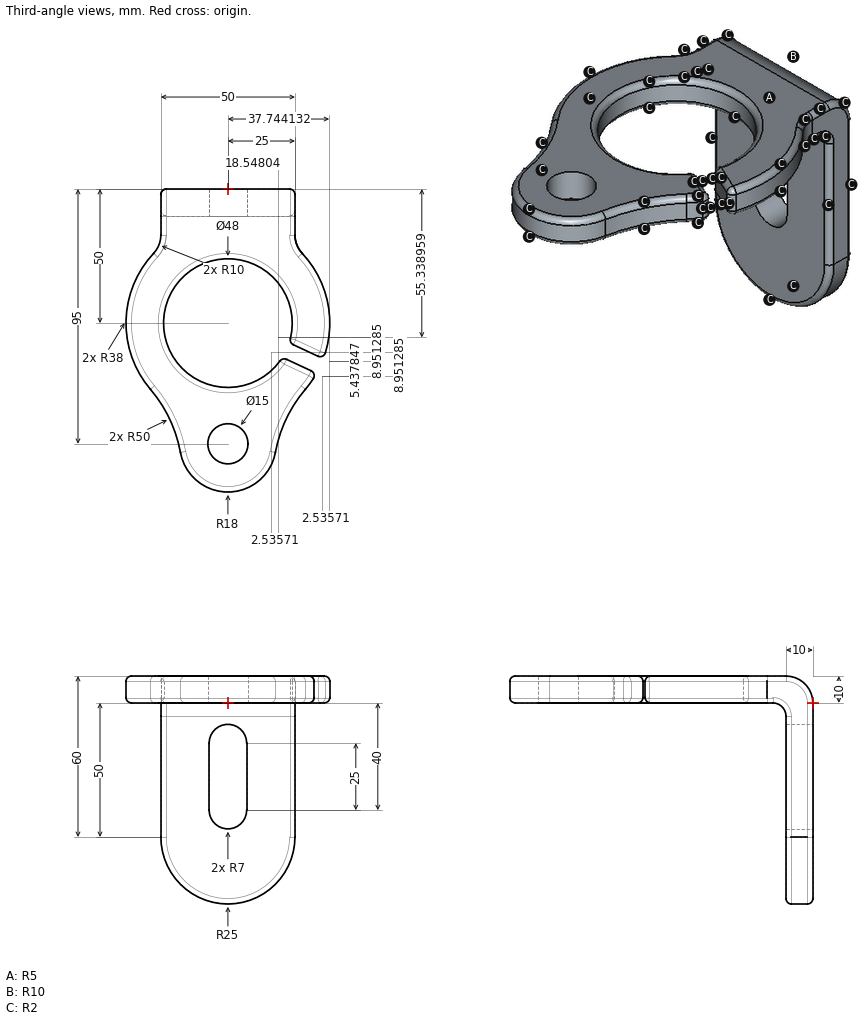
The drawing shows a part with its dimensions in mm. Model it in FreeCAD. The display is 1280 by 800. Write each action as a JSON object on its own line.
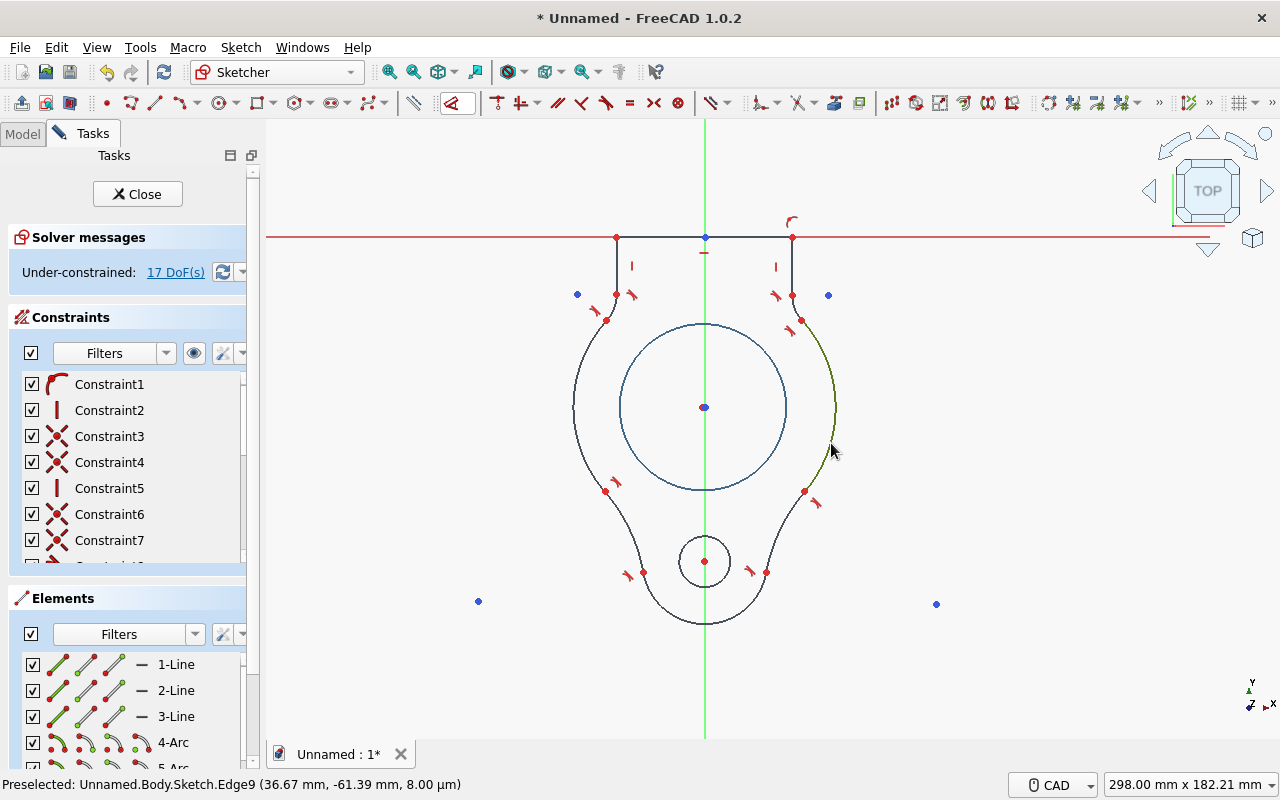
{"action": "left_click", "coordinate": [498, 104]}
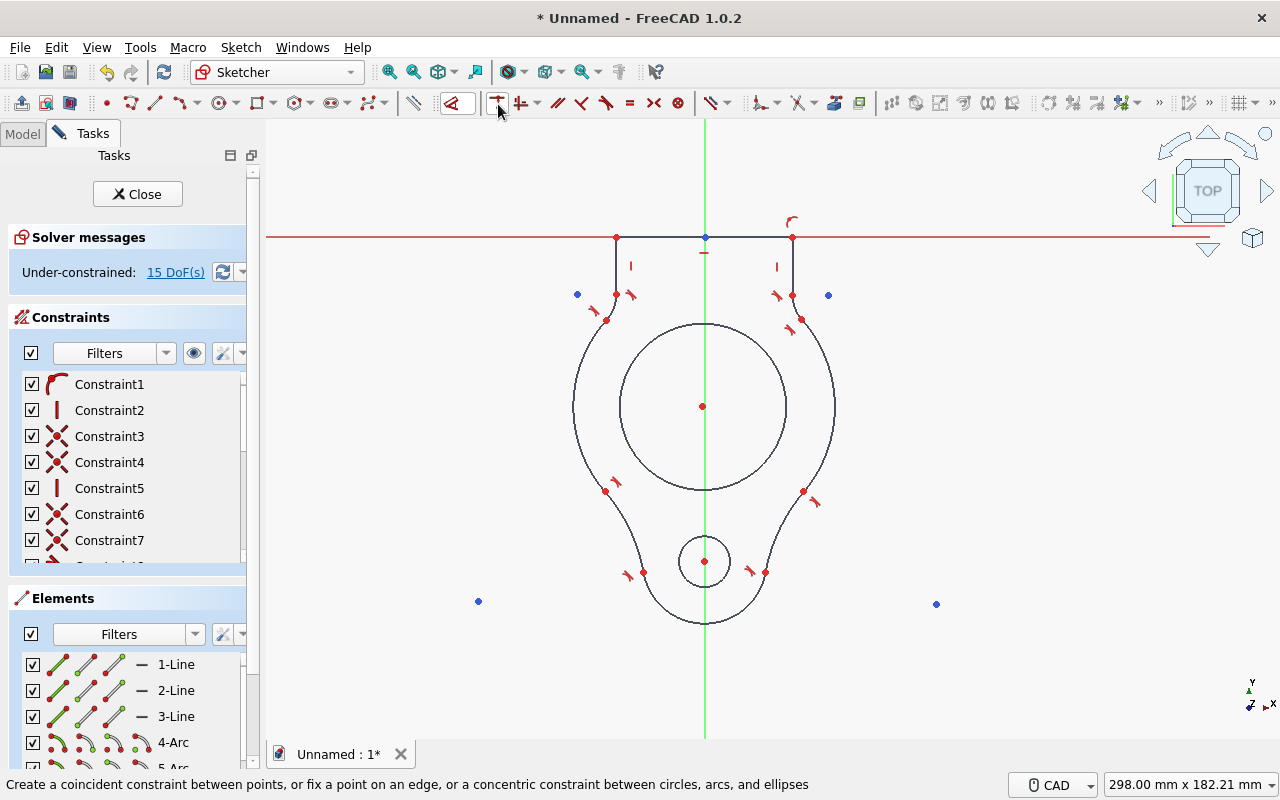
{"action": "left_click", "coordinate": [637, 546]}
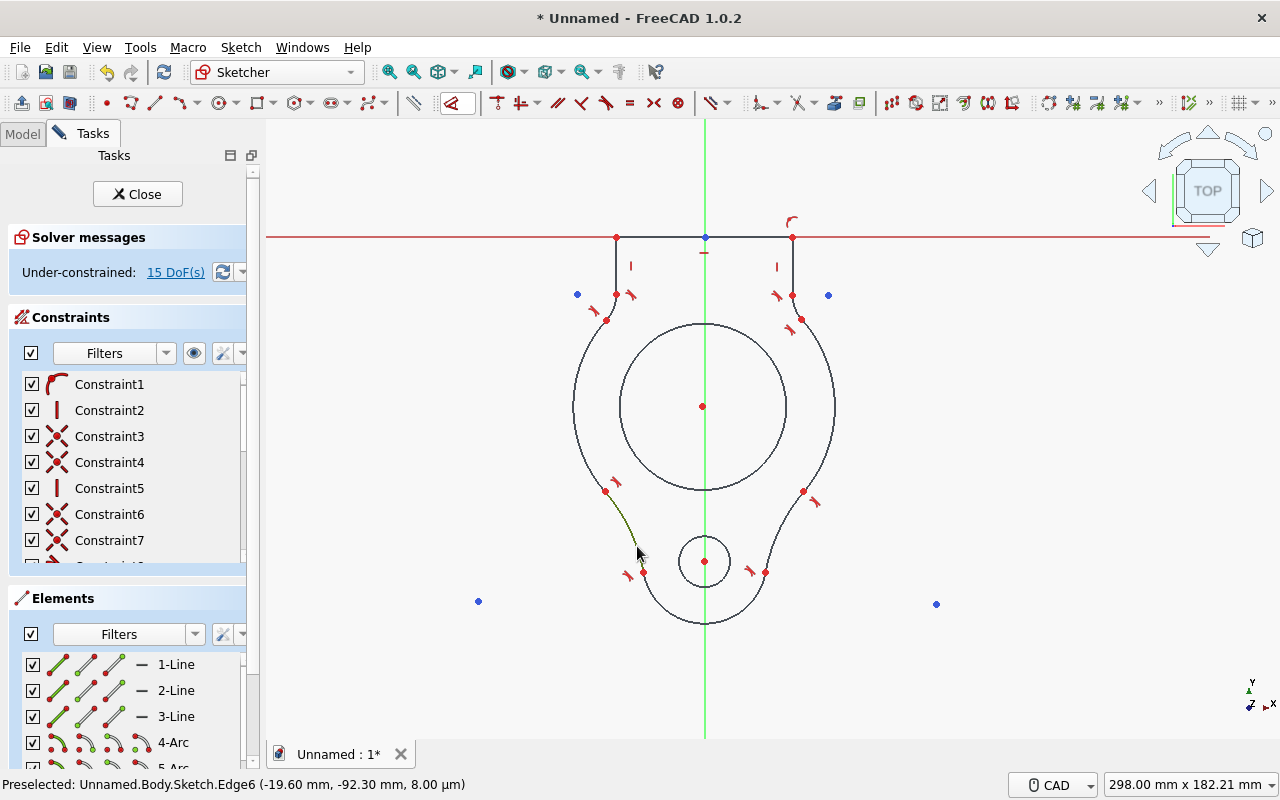
{"action": "left_click", "coordinate": [788, 514]}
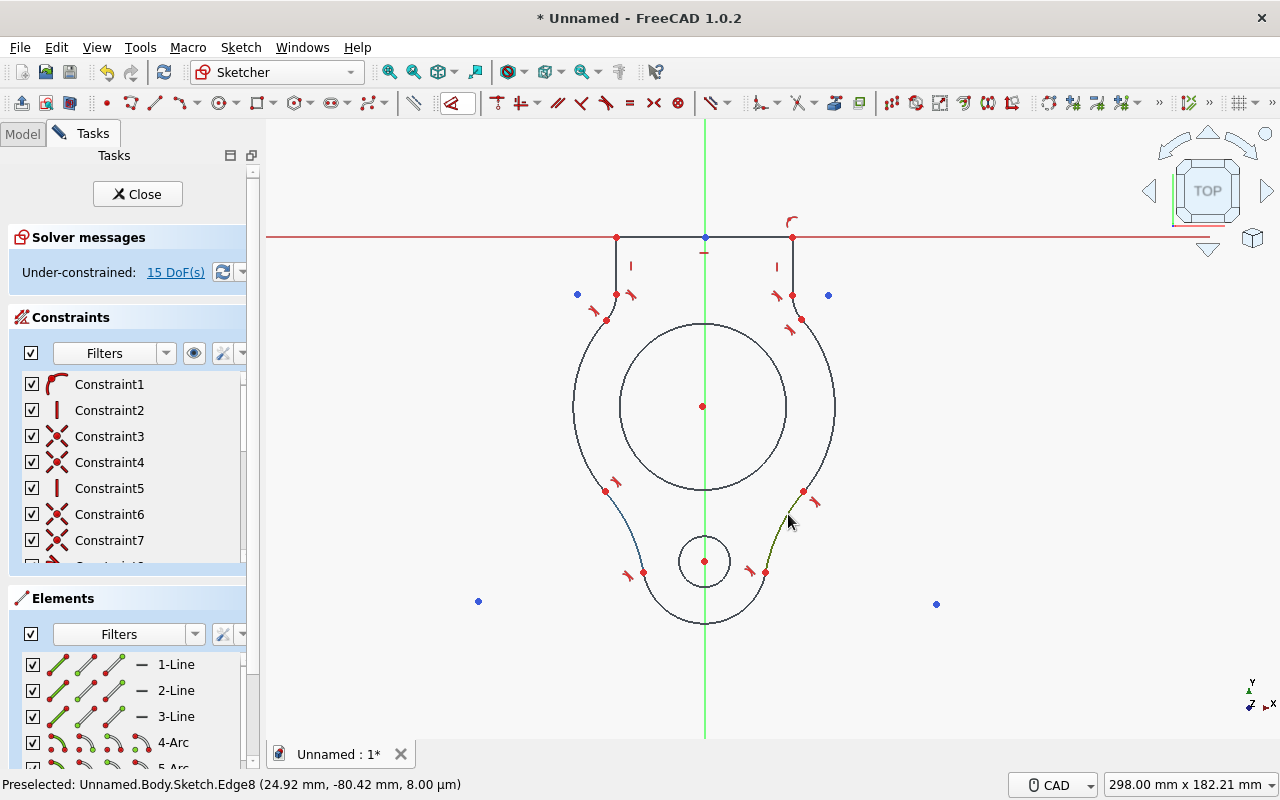
{"action": "left_click", "coordinate": [630, 104]}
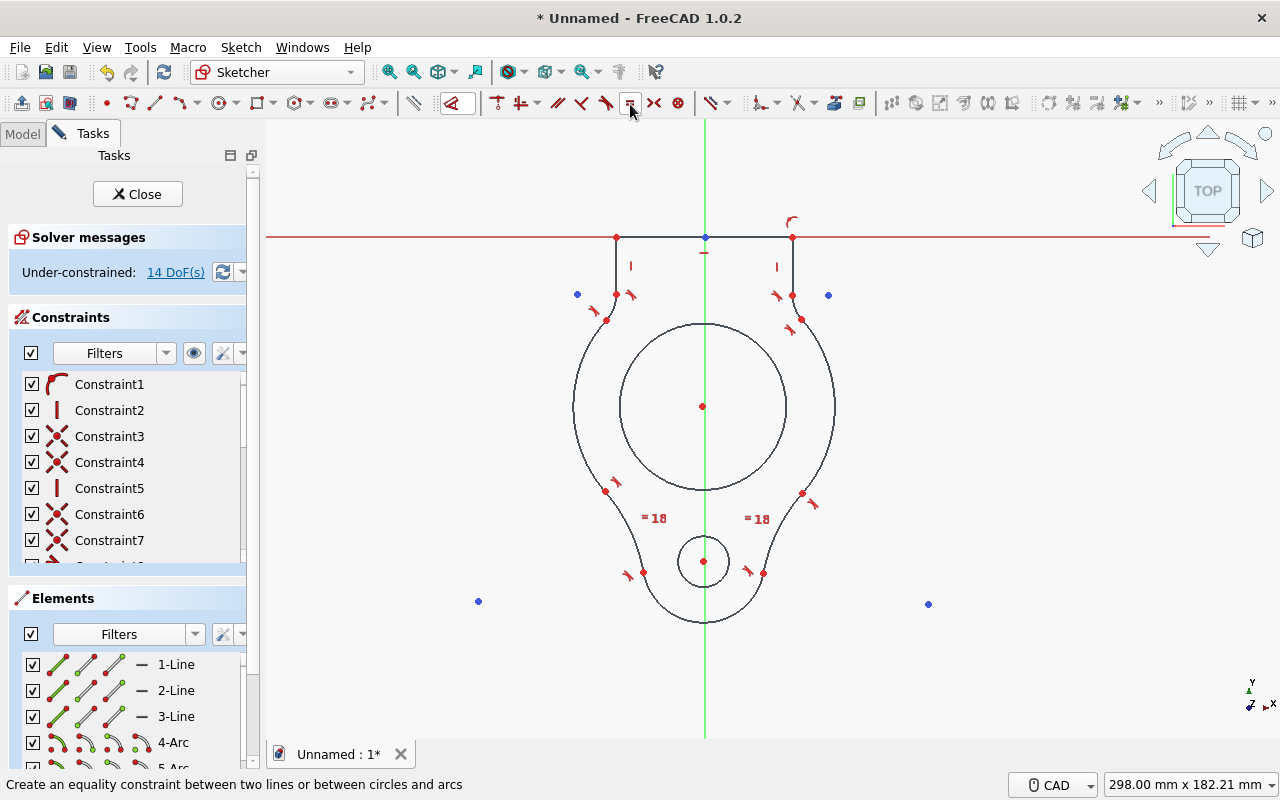
{"action": "left_click", "coordinate": [579, 369]}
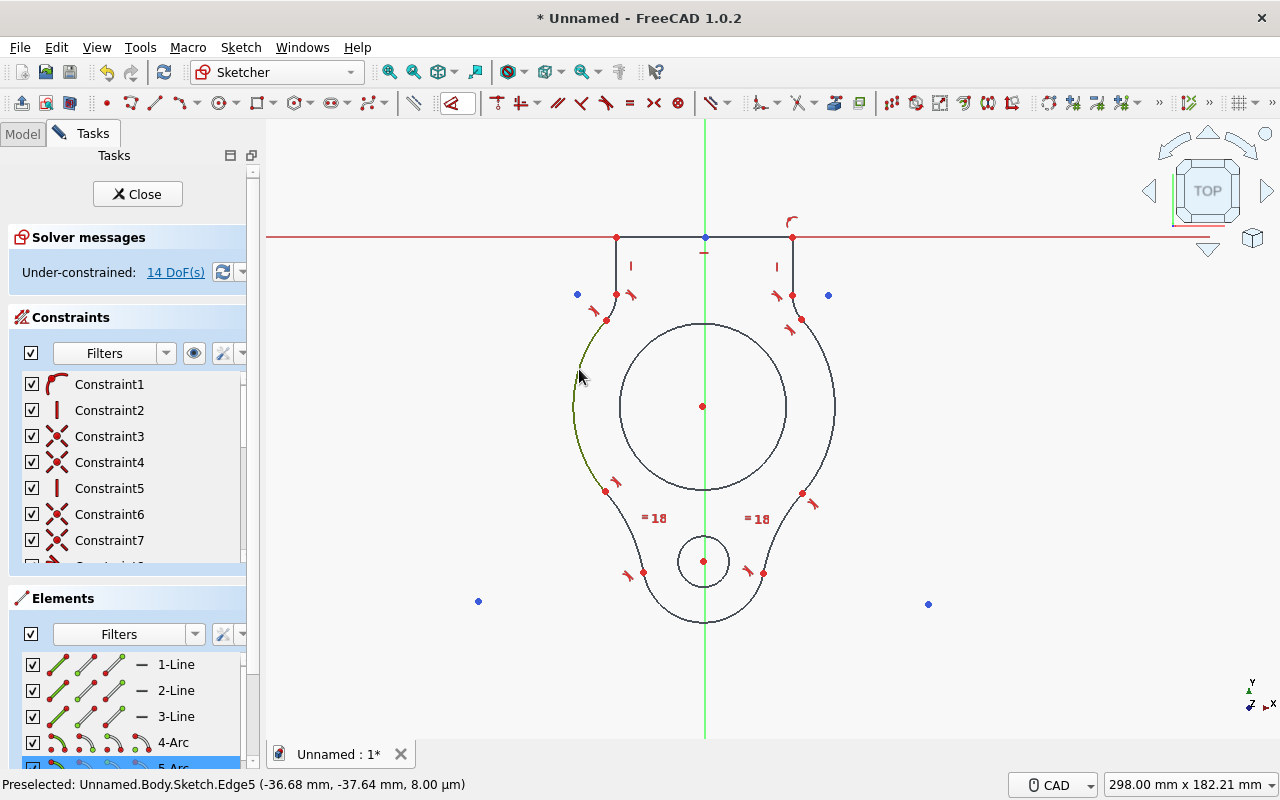
{"action": "left_click", "coordinate": [829, 444]}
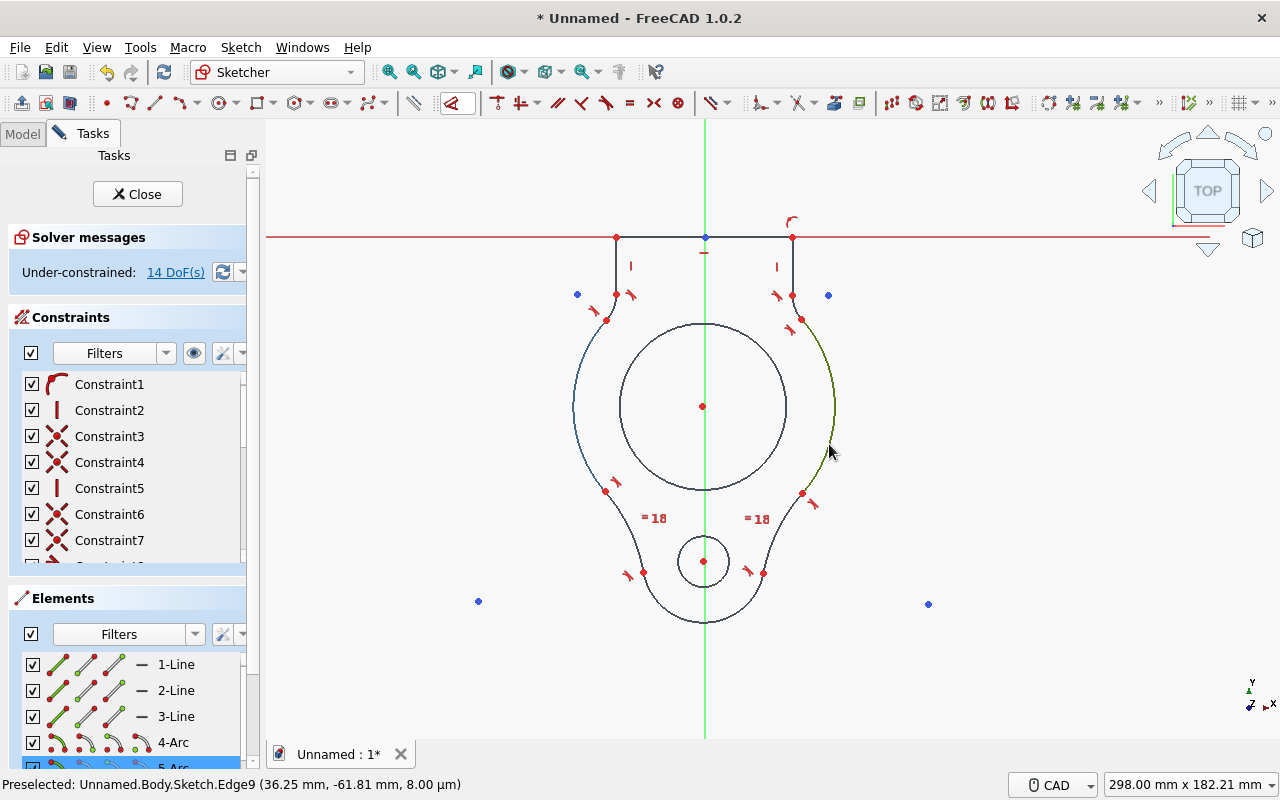
{"action": "left_click", "coordinate": [630, 104]}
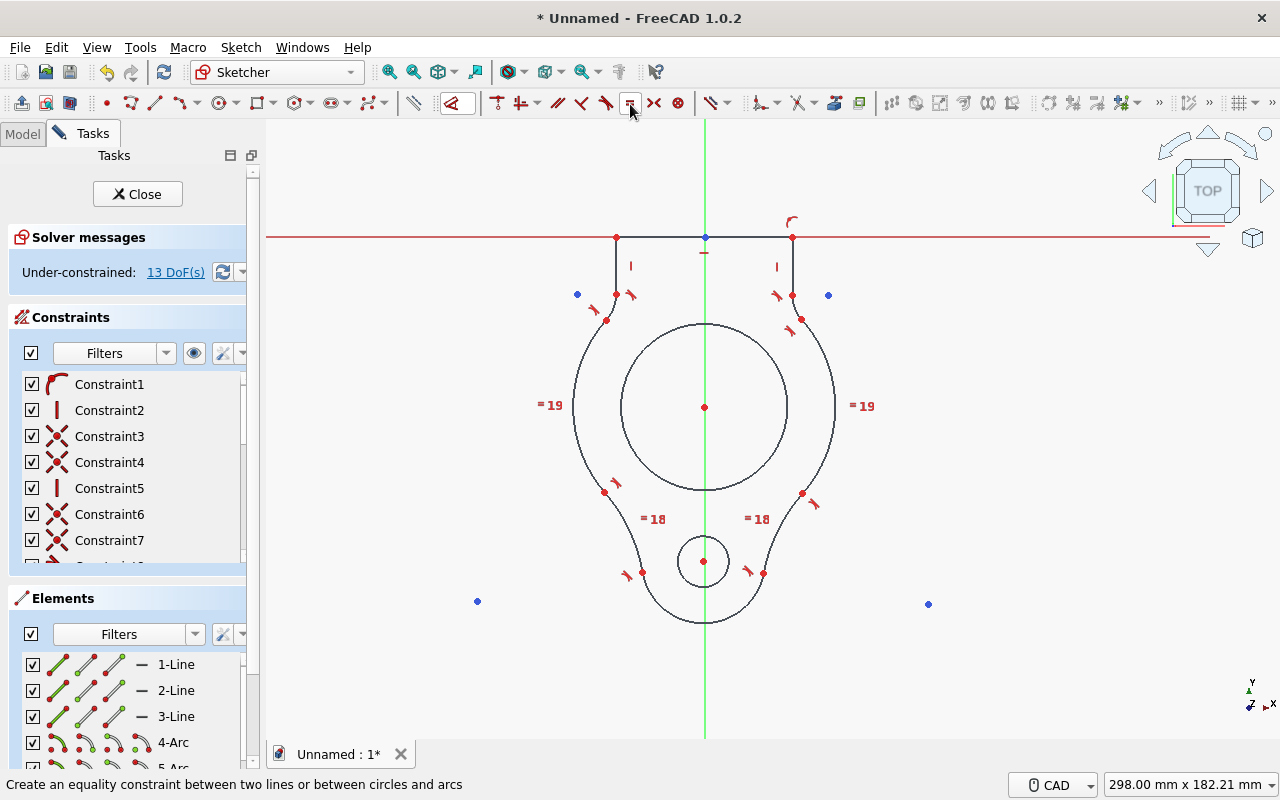
{"action": "left_click", "coordinate": [614, 308]}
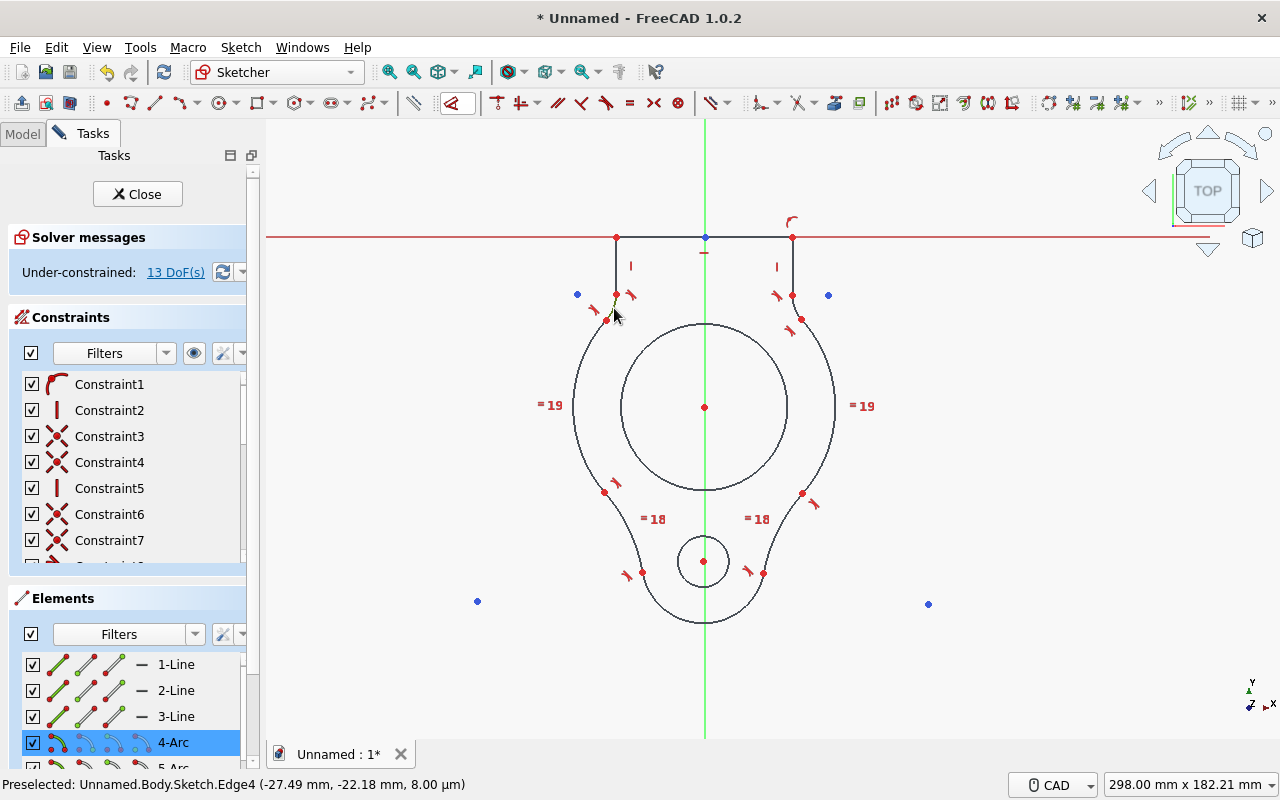
{"action": "left_click", "coordinate": [795, 309]}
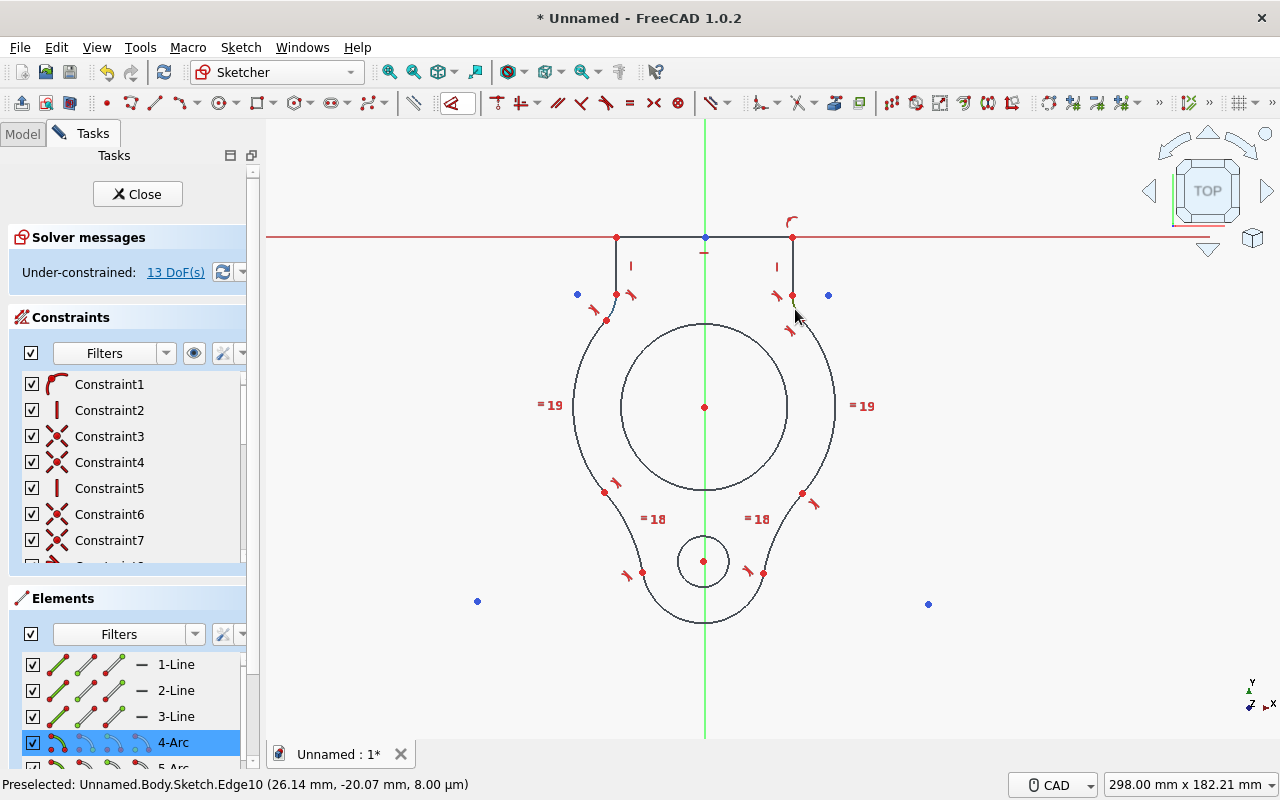
{"action": "left_click", "coordinate": [630, 104]}